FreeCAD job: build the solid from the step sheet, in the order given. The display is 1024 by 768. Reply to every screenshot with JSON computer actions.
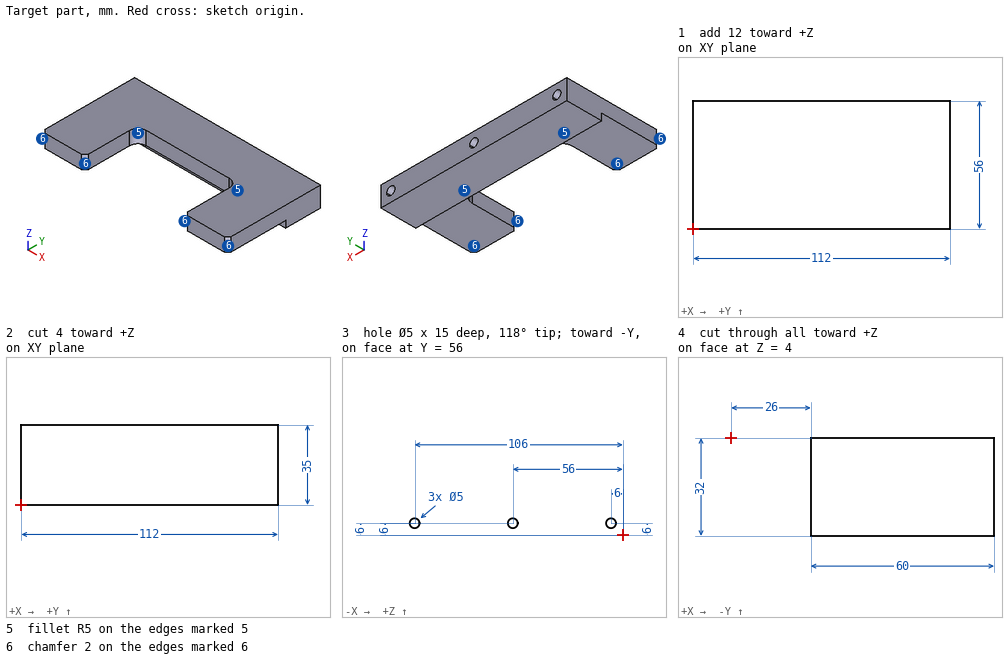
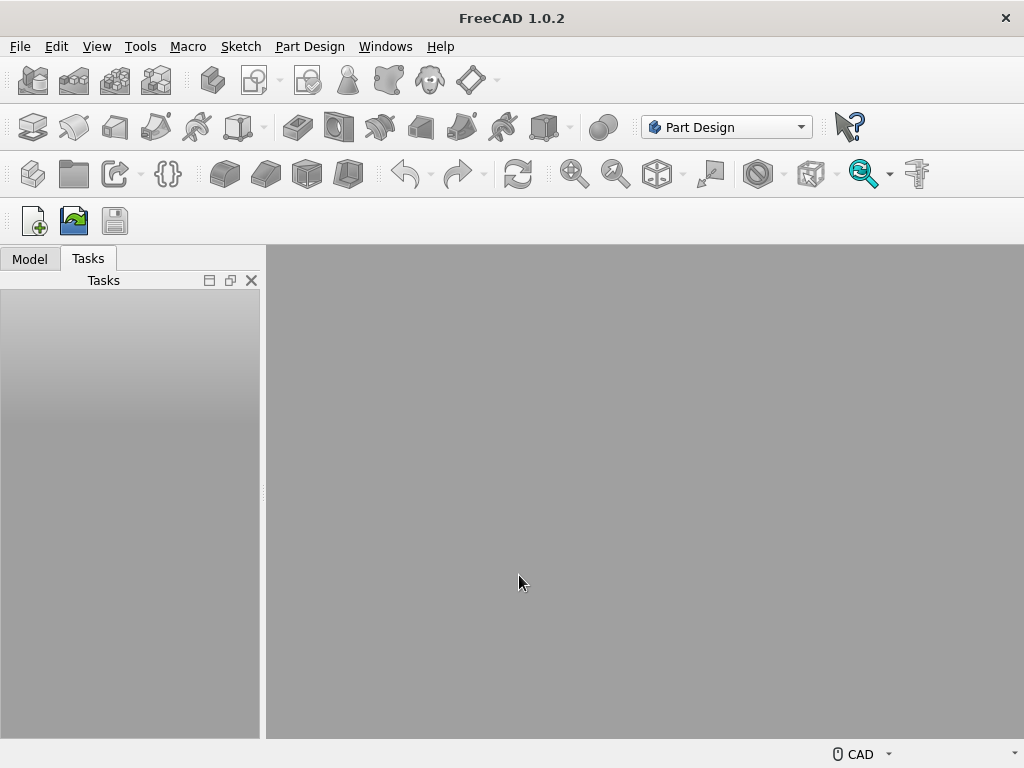
{"action": "left_click", "coordinate": [33, 222]}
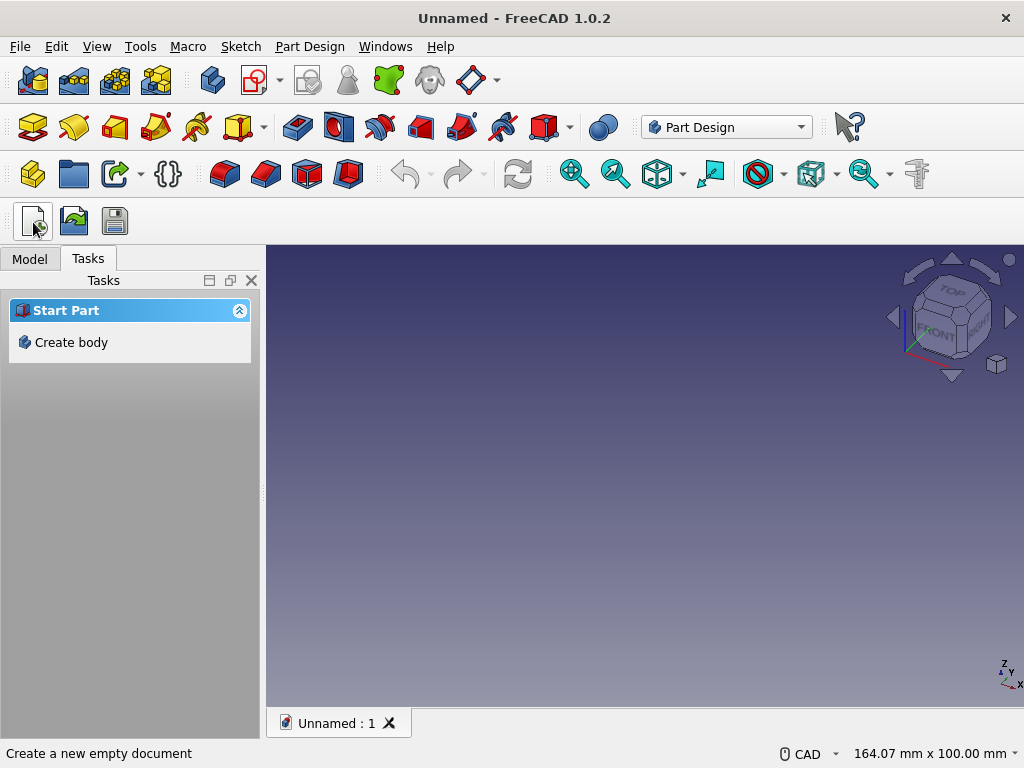
{"action": "left_click", "coordinate": [254, 80]}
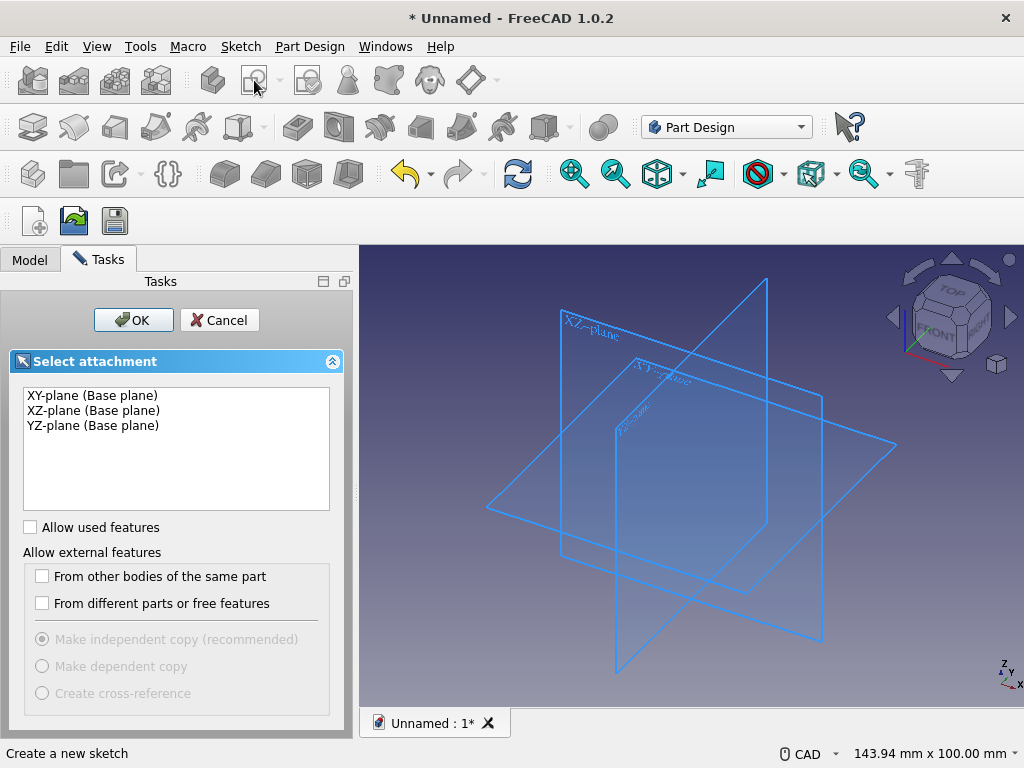
{"action": "left_click", "coordinate": [84, 396]}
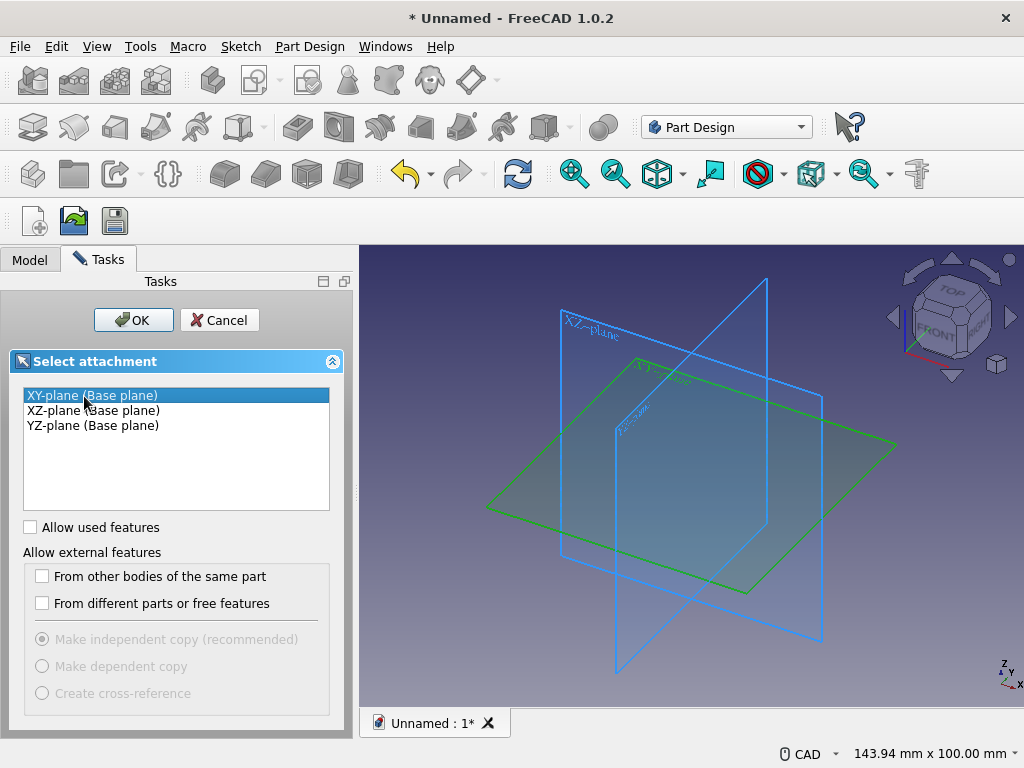
{"action": "left_click", "coordinate": [134, 320]}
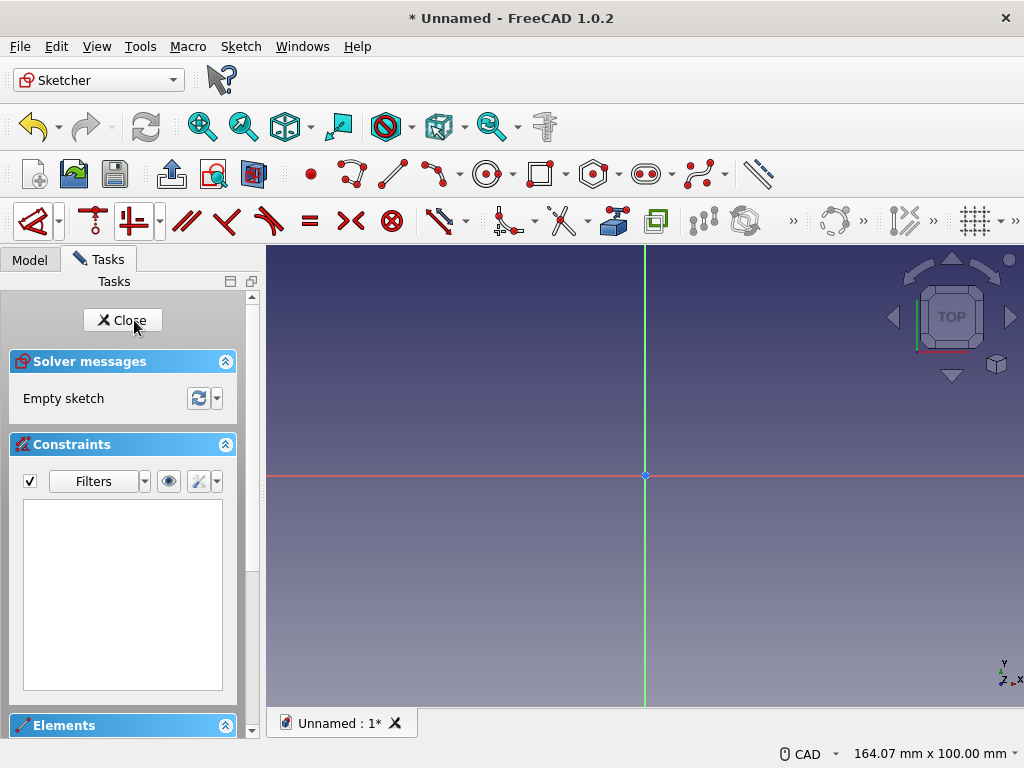
{"action": "scroll", "coordinate": [294, 633], "scroll_direction": "down", "scroll_amount": 3}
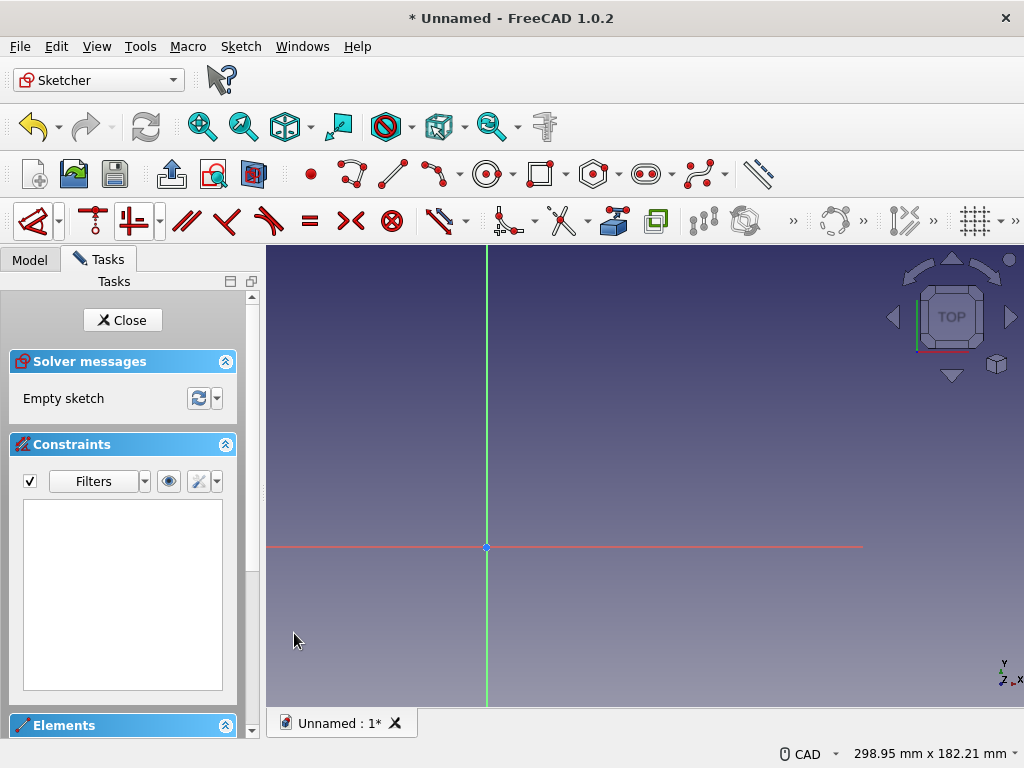
{"action": "scroll", "coordinate": [735, 477], "scroll_direction": "up", "scroll_amount": 2}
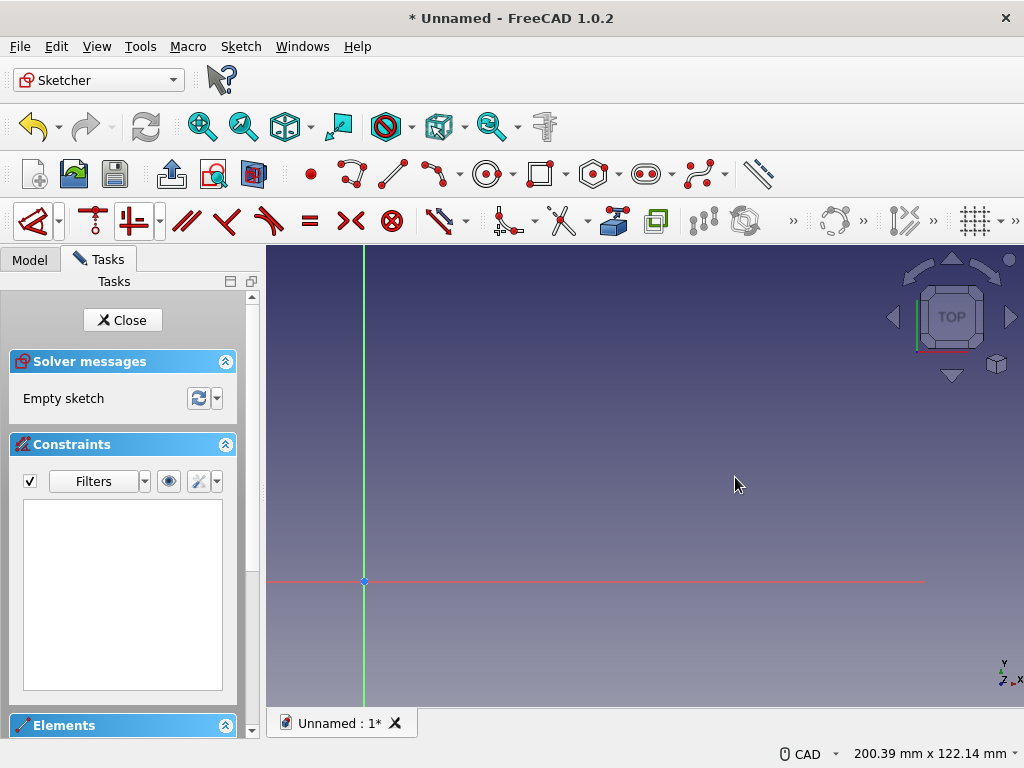
{"action": "left_click", "coordinate": [540, 174]}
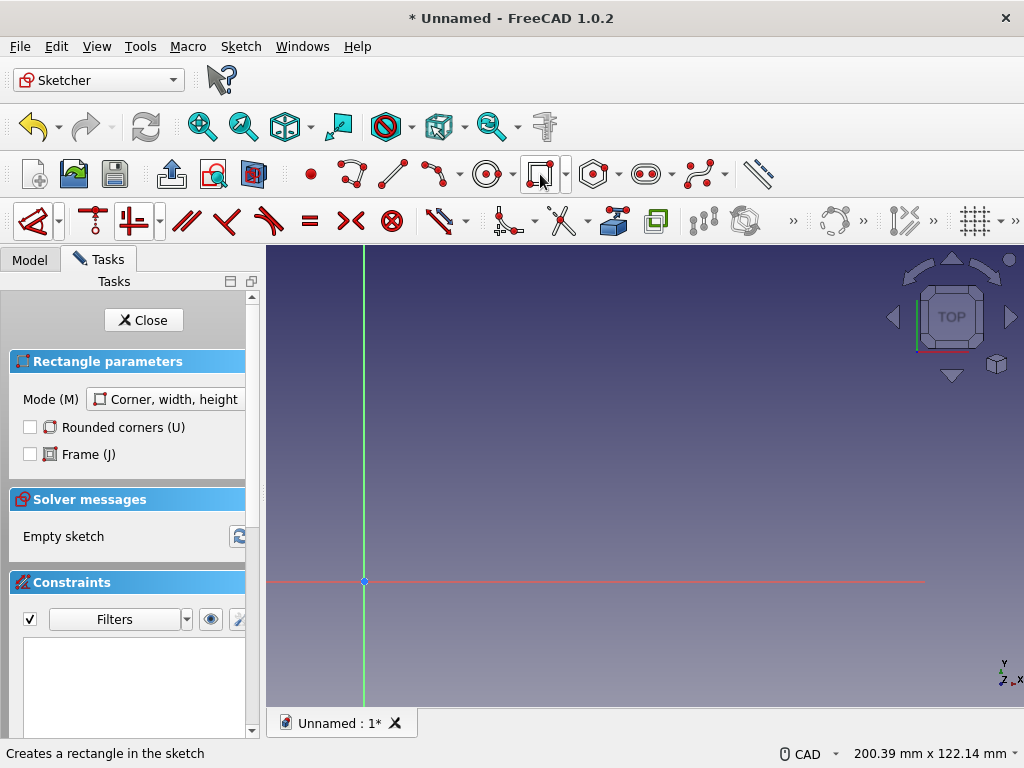
{"action": "left_click", "coordinate": [364, 582]}
{"action": "left_click", "coordinate": [788, 370]}
{"action": "key", "text": "Escape"}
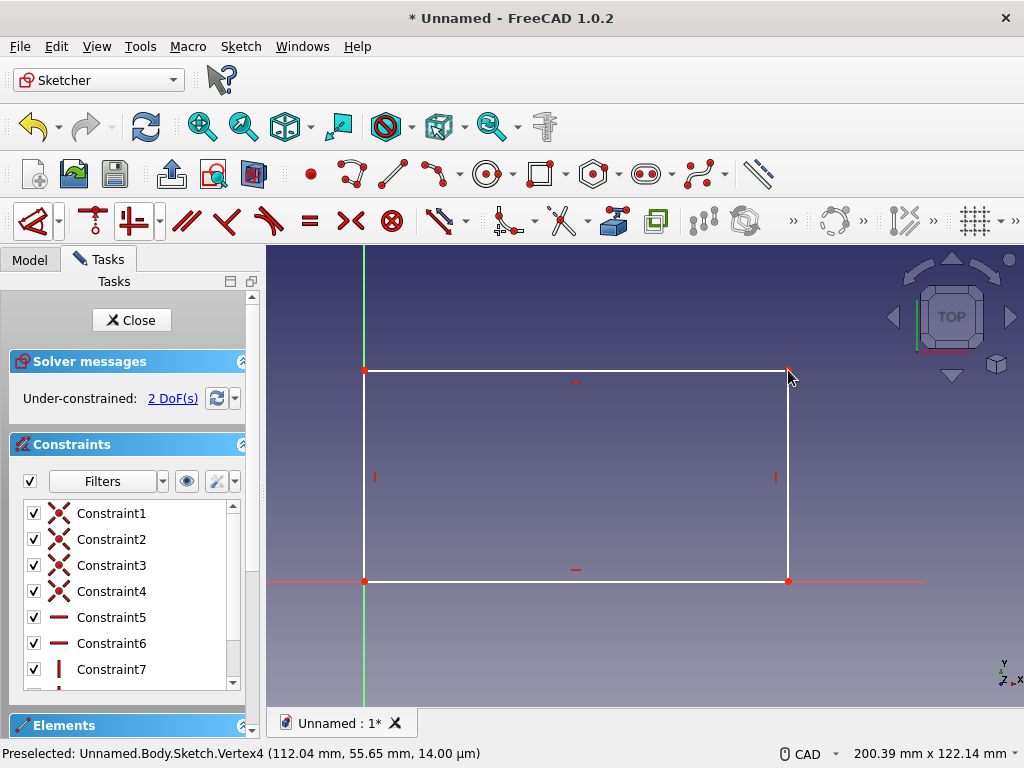
{"action": "left_click", "coordinate": [32, 222]}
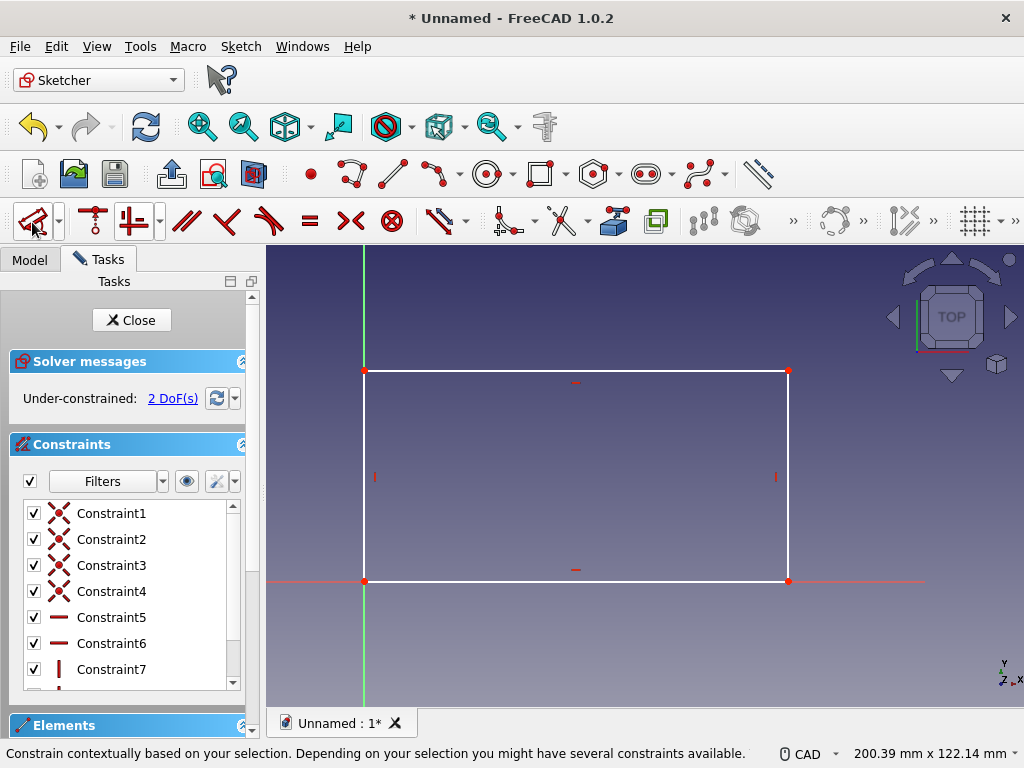
{"action": "left_click", "coordinate": [788, 518]}
{"action": "left_click", "coordinate": [822, 476]}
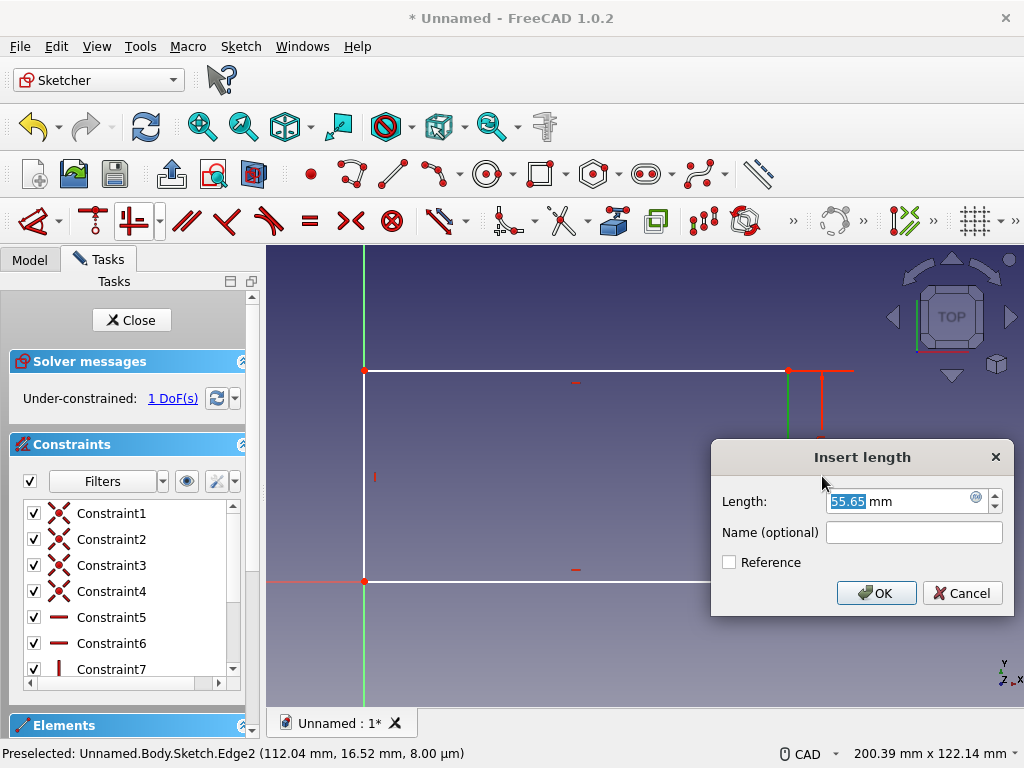
{"action": "type", "text": "56"}
{"action": "key", "text": "Return"}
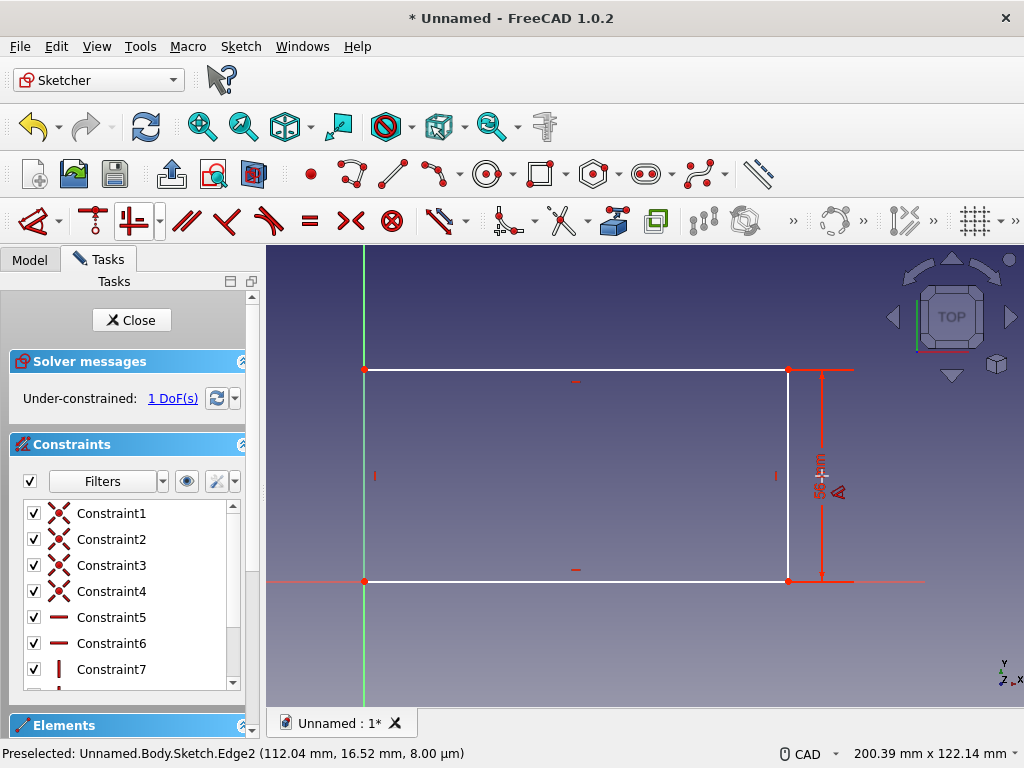
{"action": "left_click", "coordinate": [491, 582]}
{"action": "left_click", "coordinate": [576, 616]}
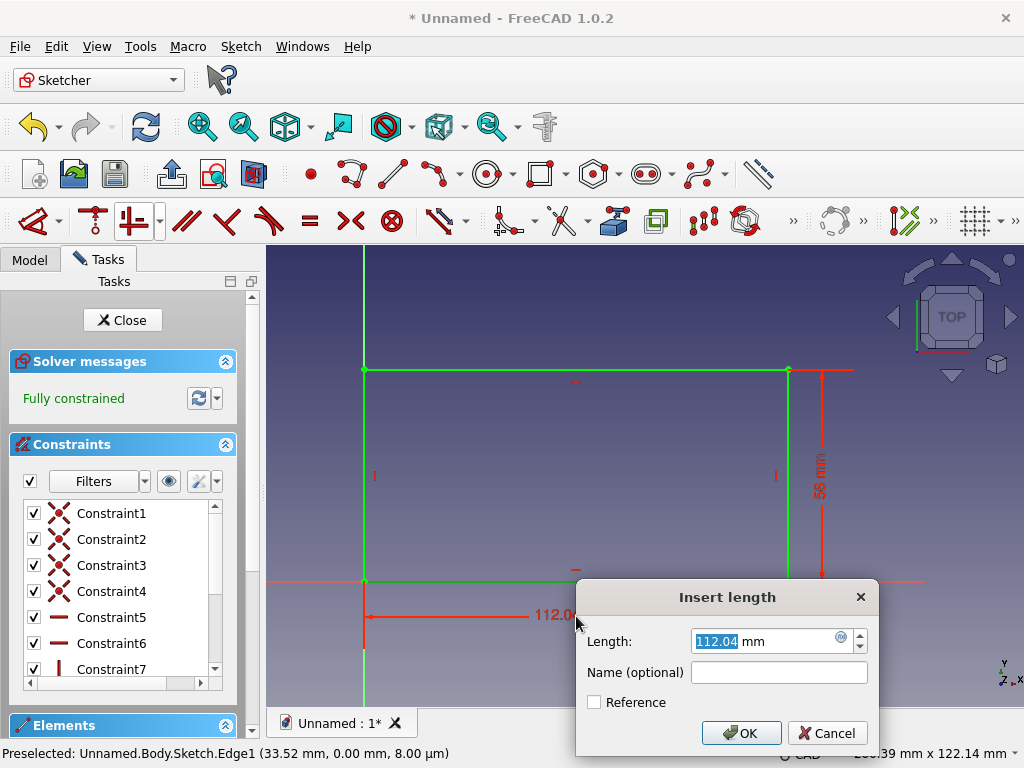
{"action": "type", "text": "112"}
{"action": "key", "text": "Return"}
{"action": "key", "text": "Escape"}